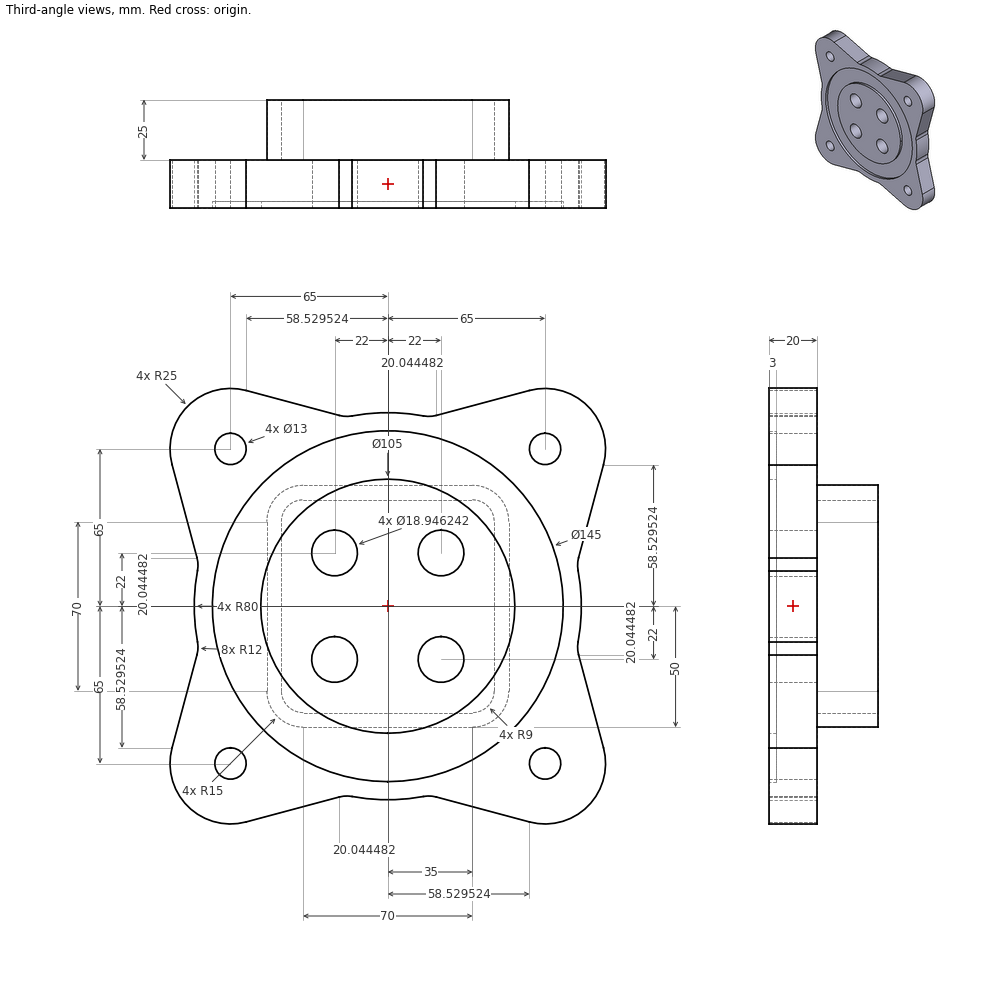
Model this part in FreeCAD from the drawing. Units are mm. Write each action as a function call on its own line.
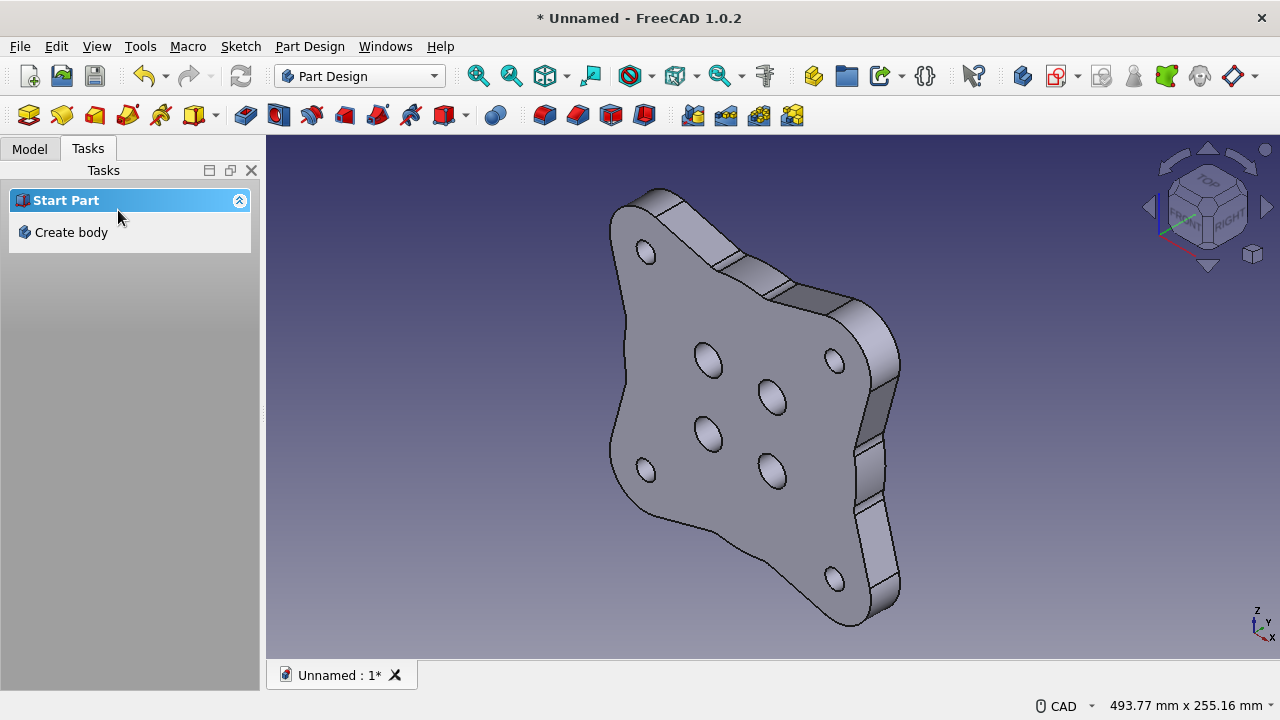
click(740, 329)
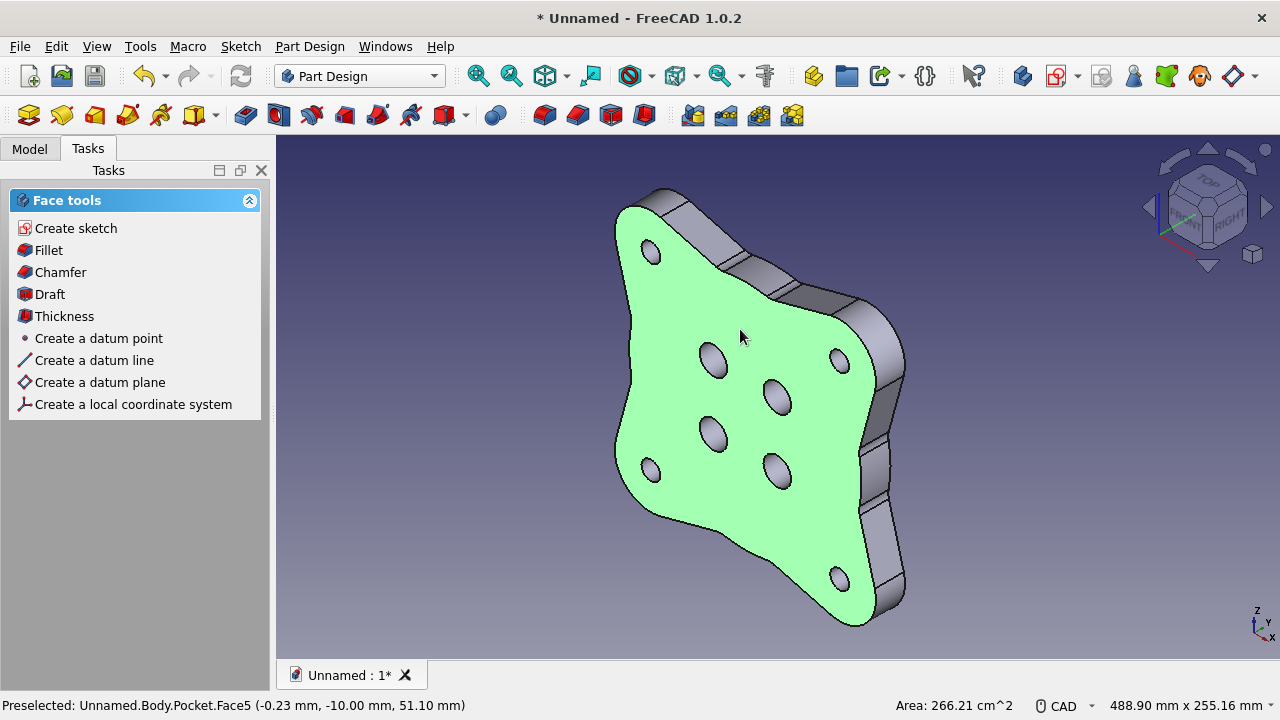
click(1056, 76)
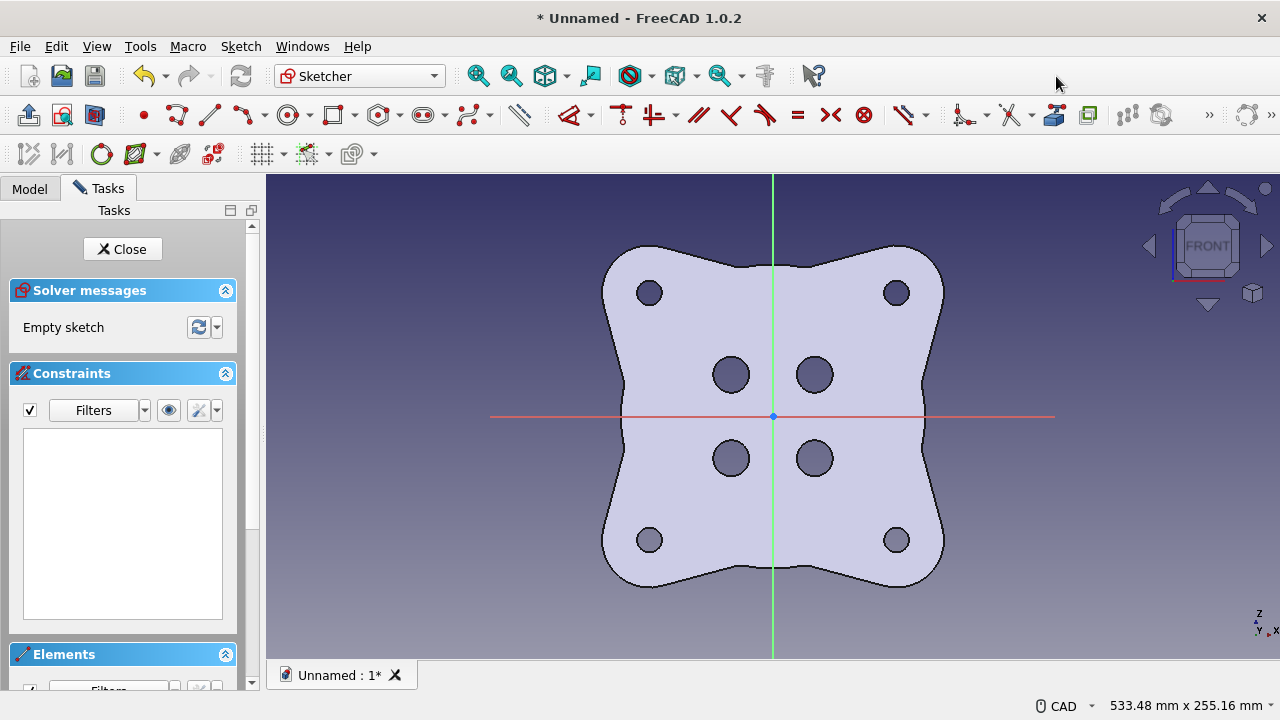
click(288, 116)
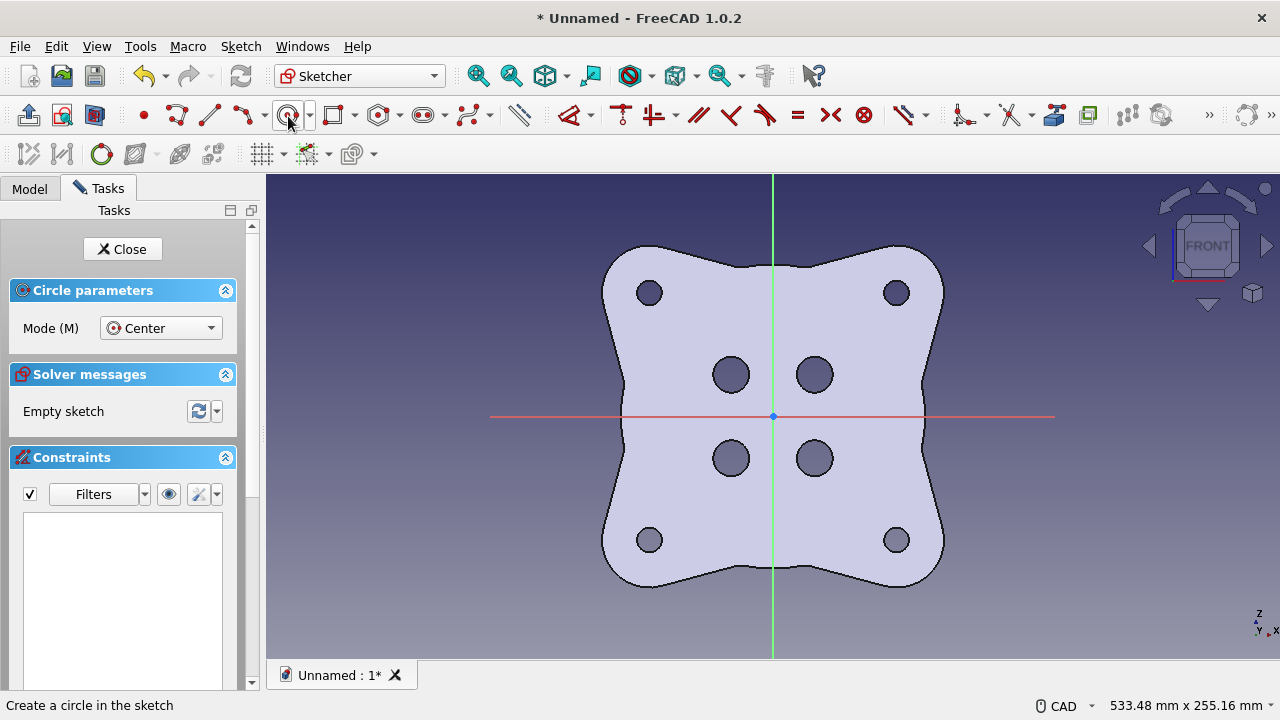
click(773, 417)
move(870, 319)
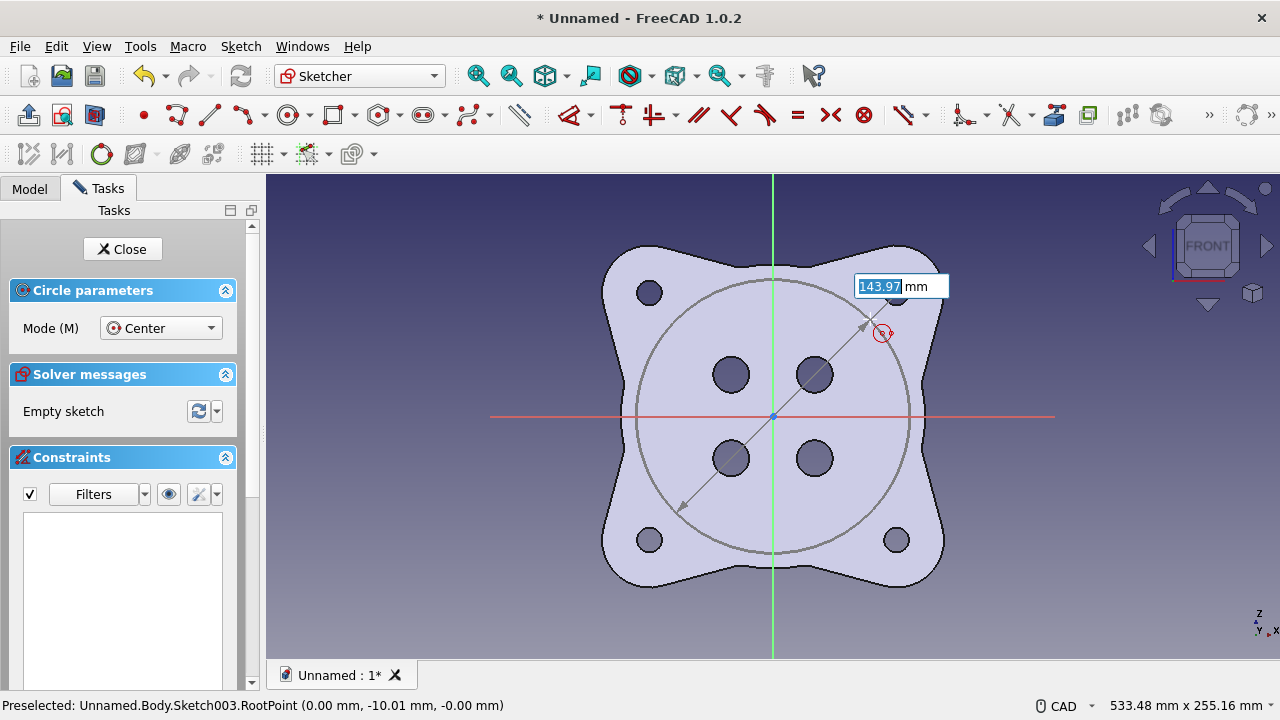
text(145)
key(Return)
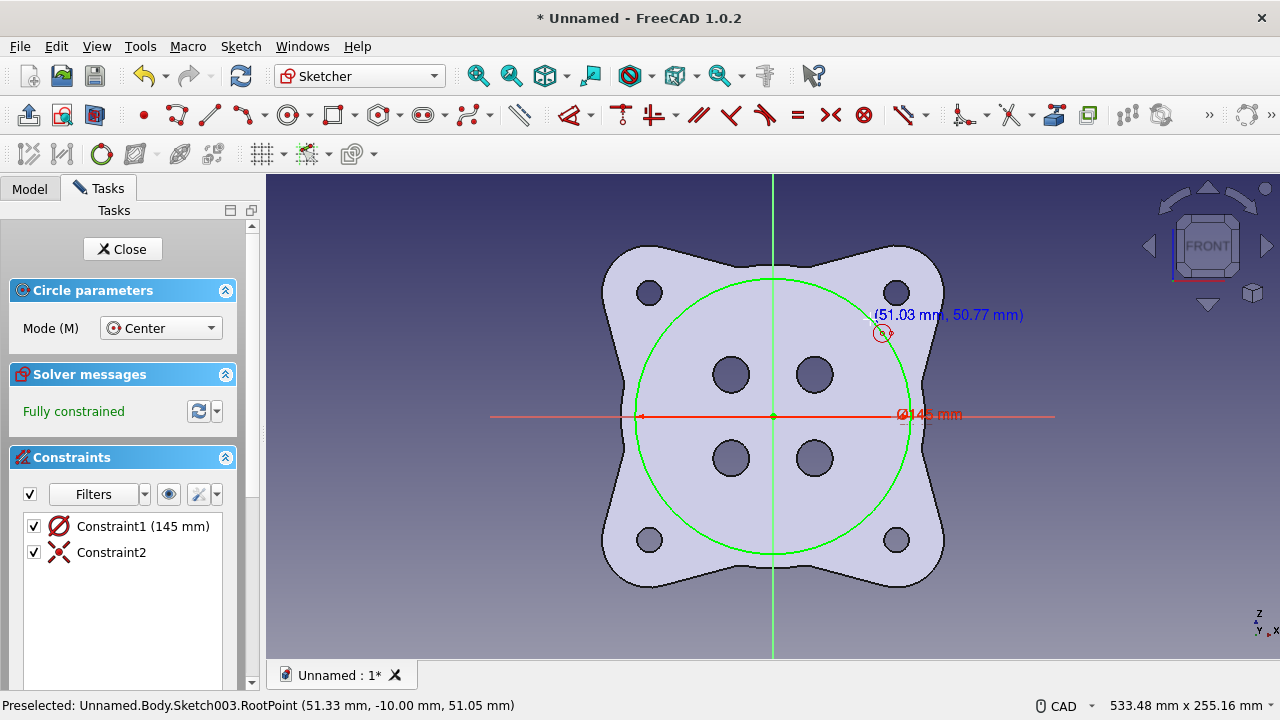
click(773, 417)
move(844, 346)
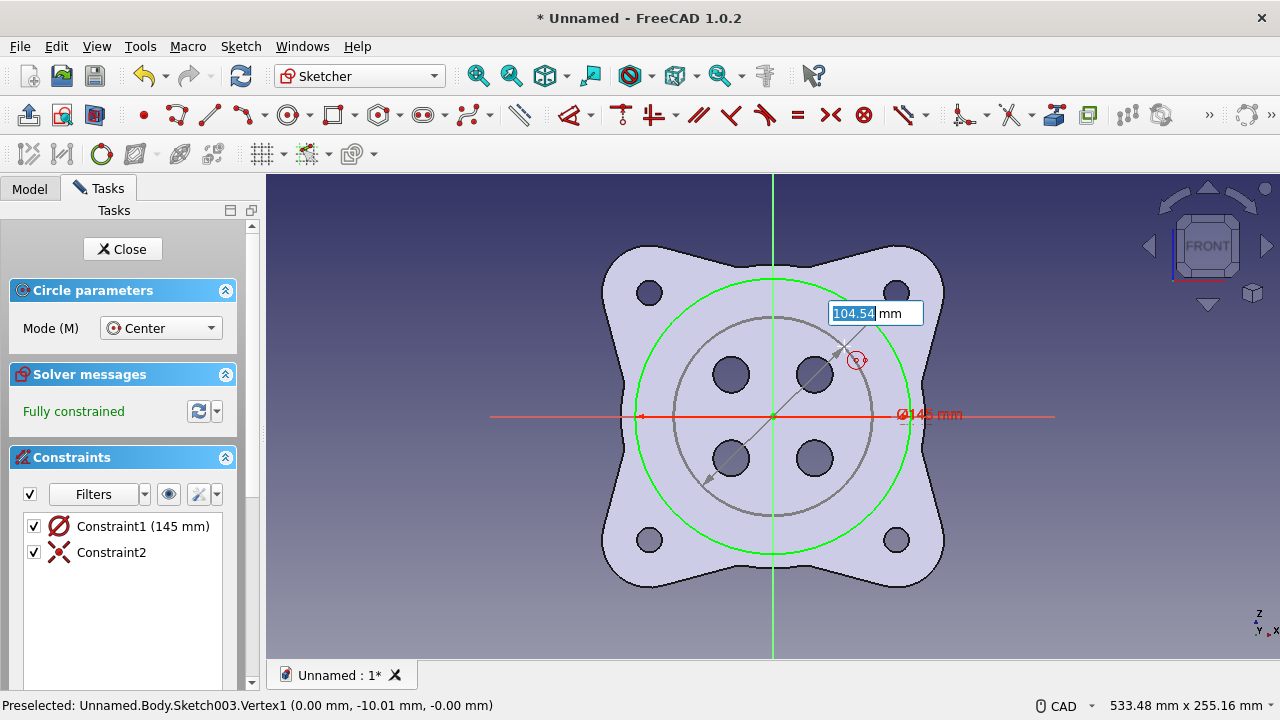
text(105)
key(Return)
key(Escape)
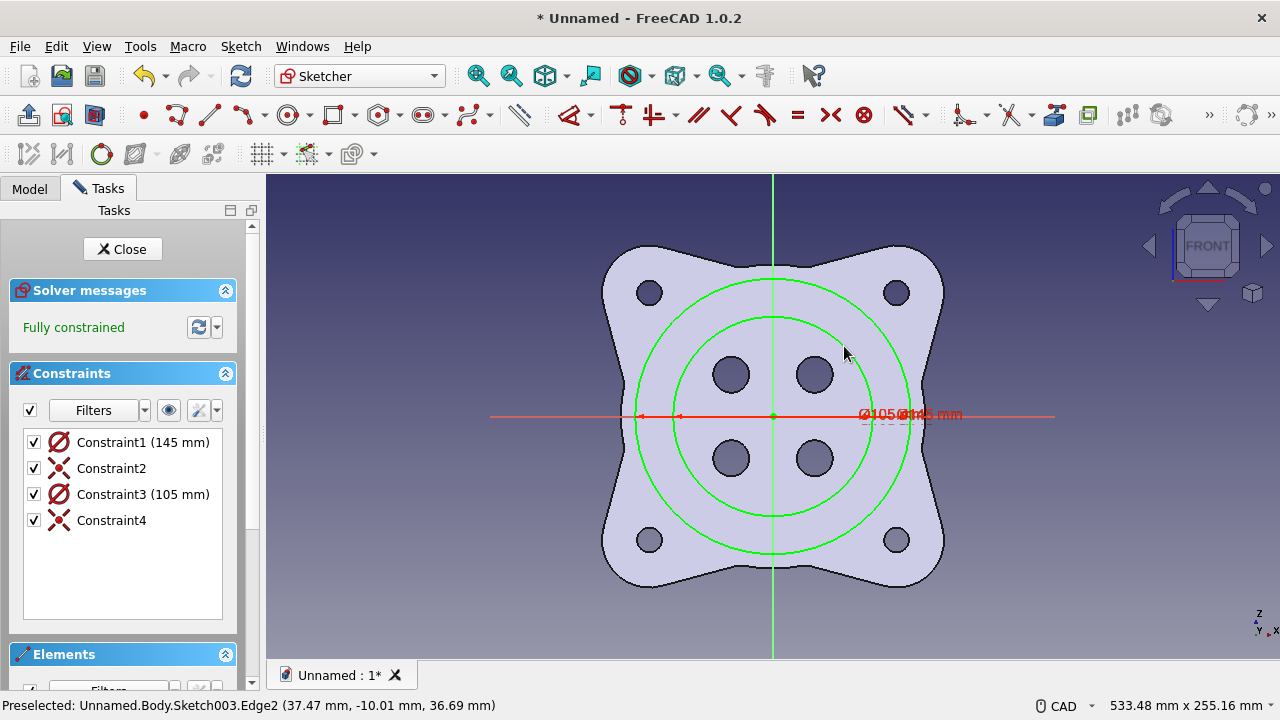
click(123, 249)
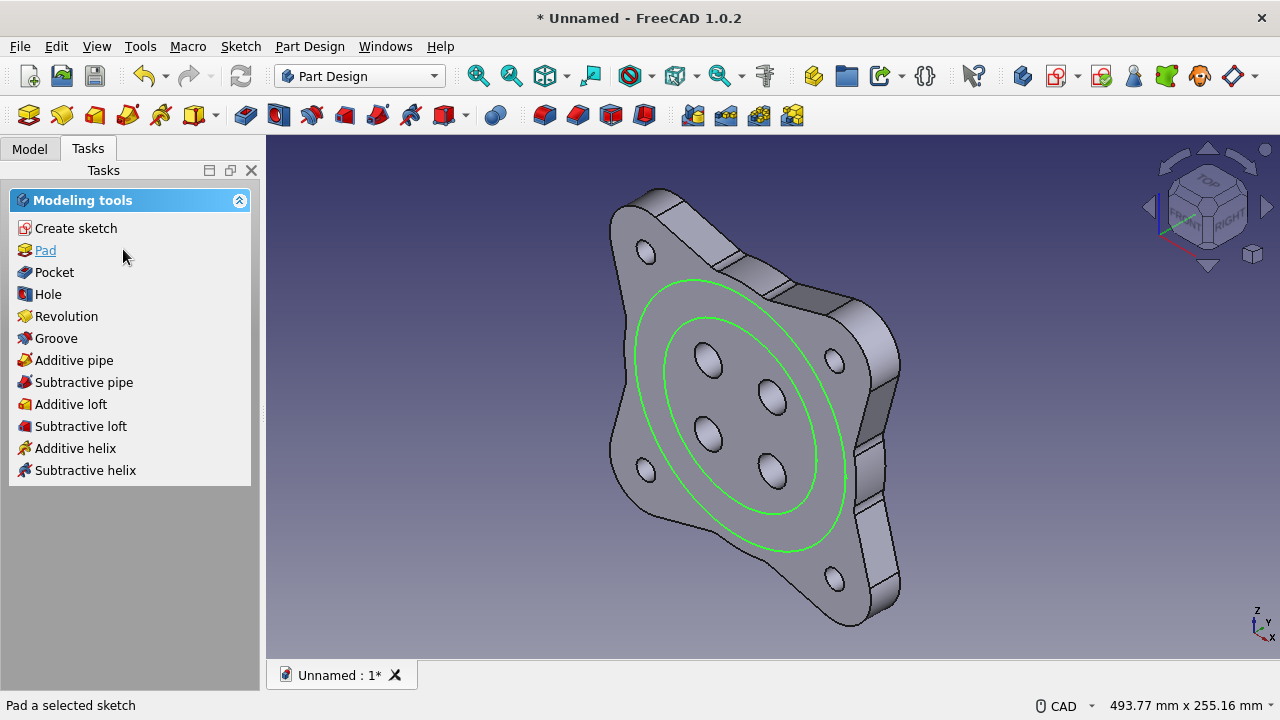
click(246, 116)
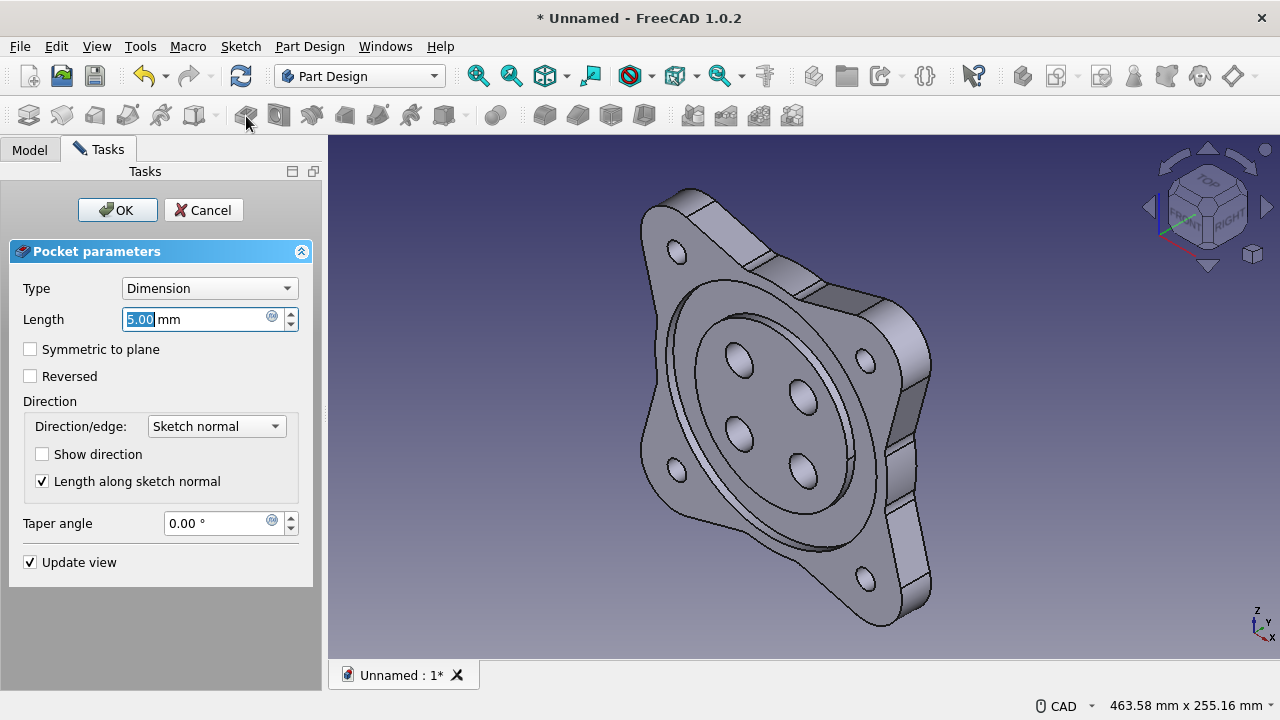
click(210, 288)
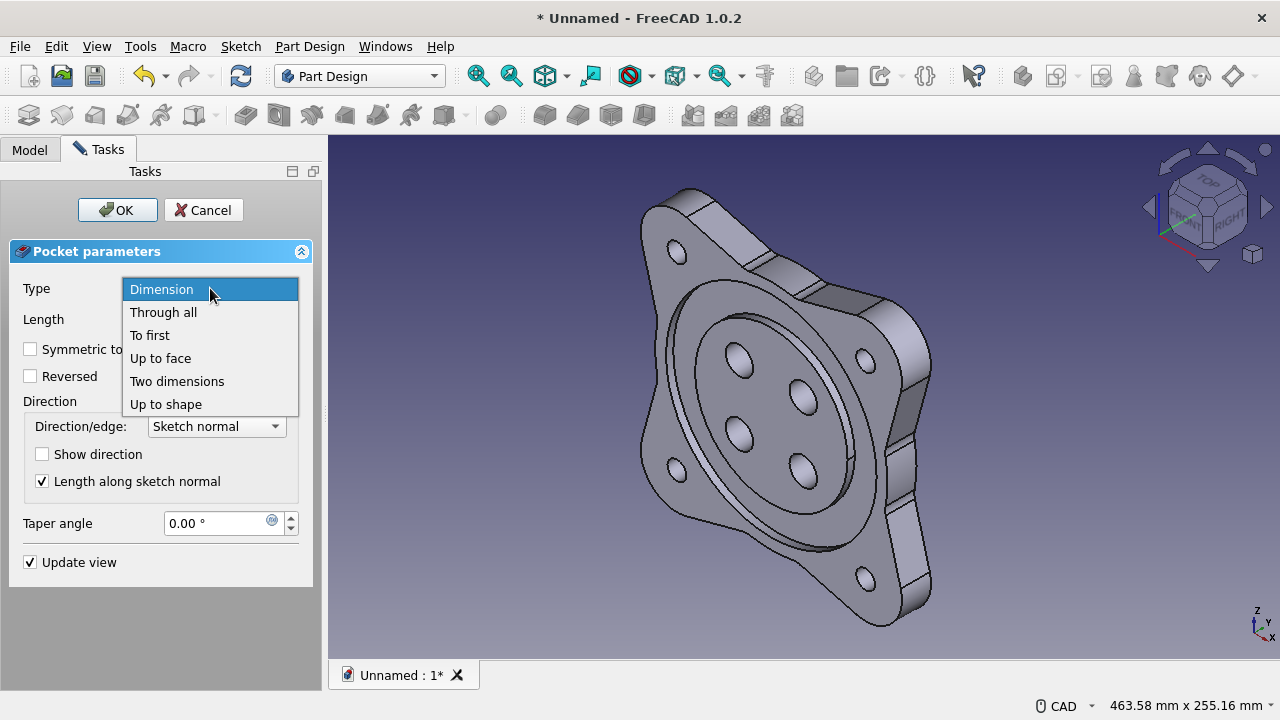
click(208, 382)